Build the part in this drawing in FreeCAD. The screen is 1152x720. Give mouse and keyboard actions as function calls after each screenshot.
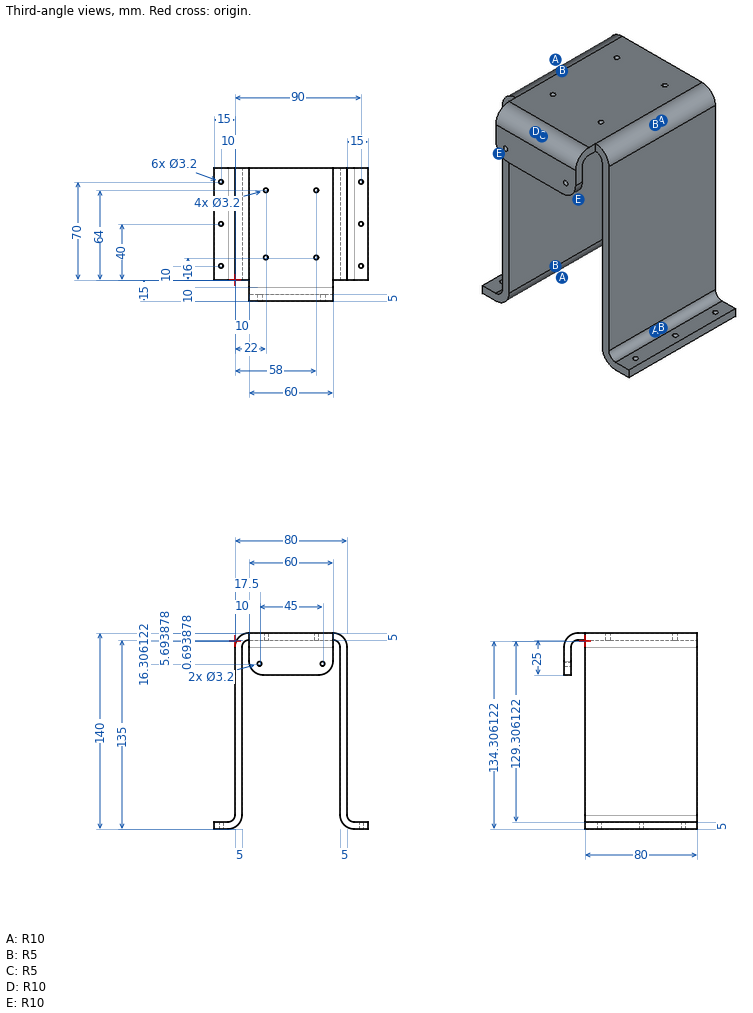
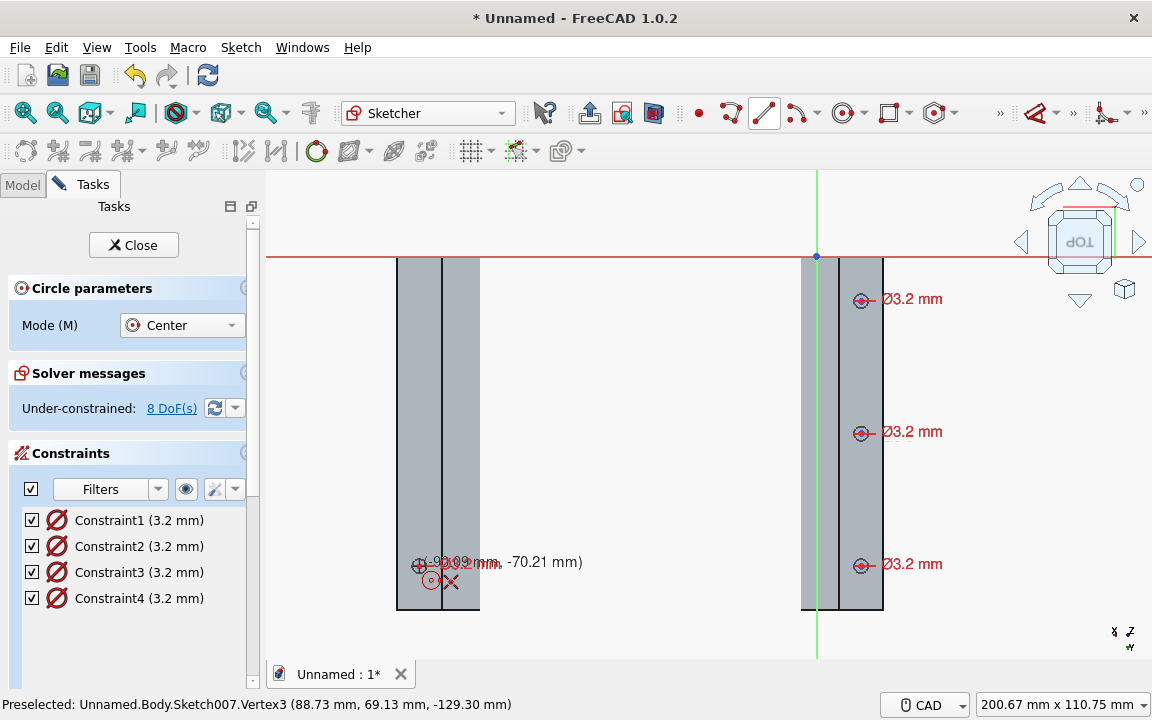
scroll(420, 433, up, 6)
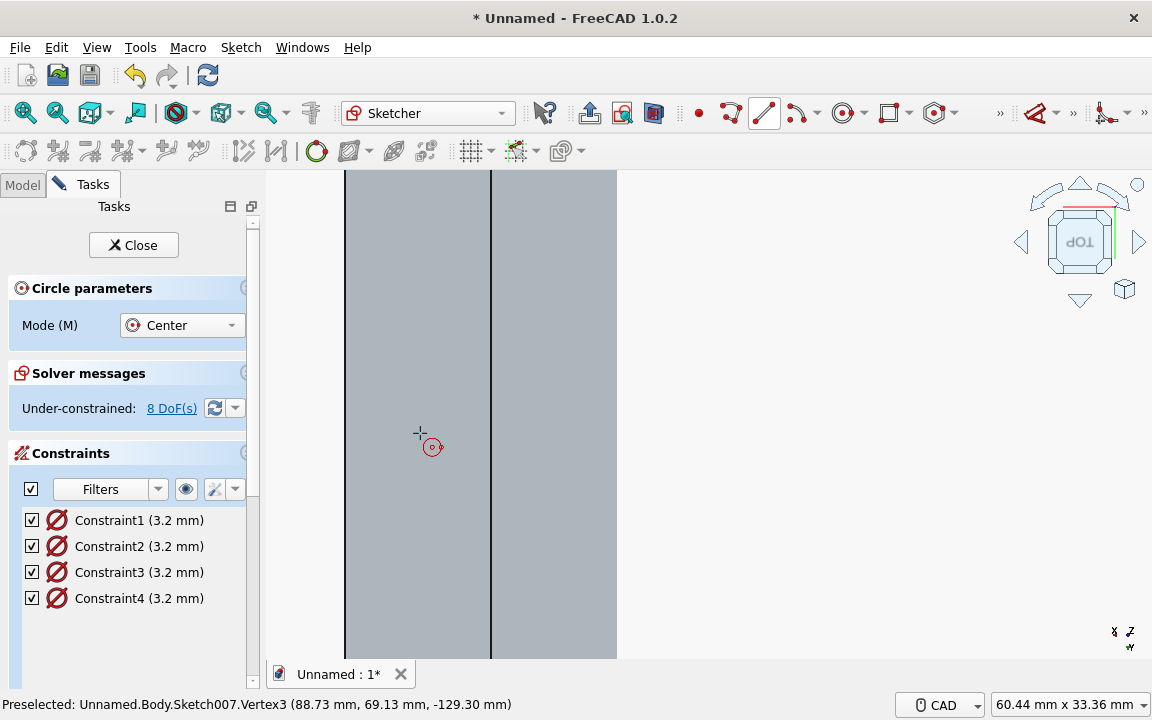
click(418, 433)
move(435, 417)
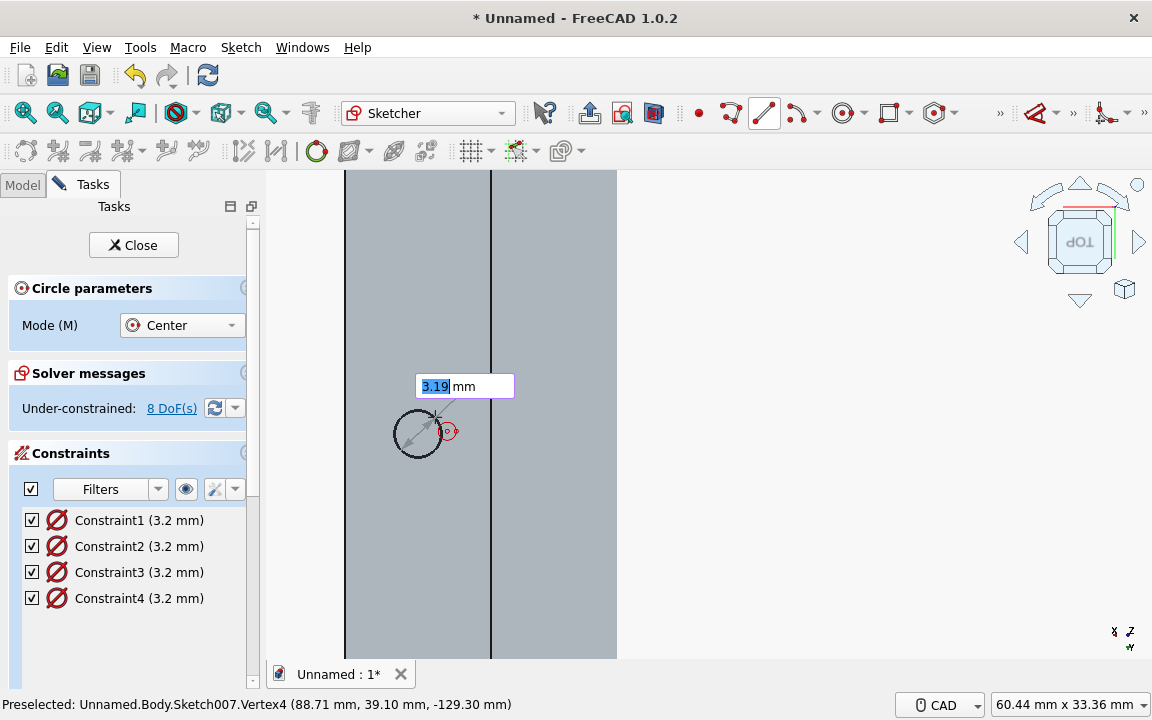
text(3.2)
key(Return)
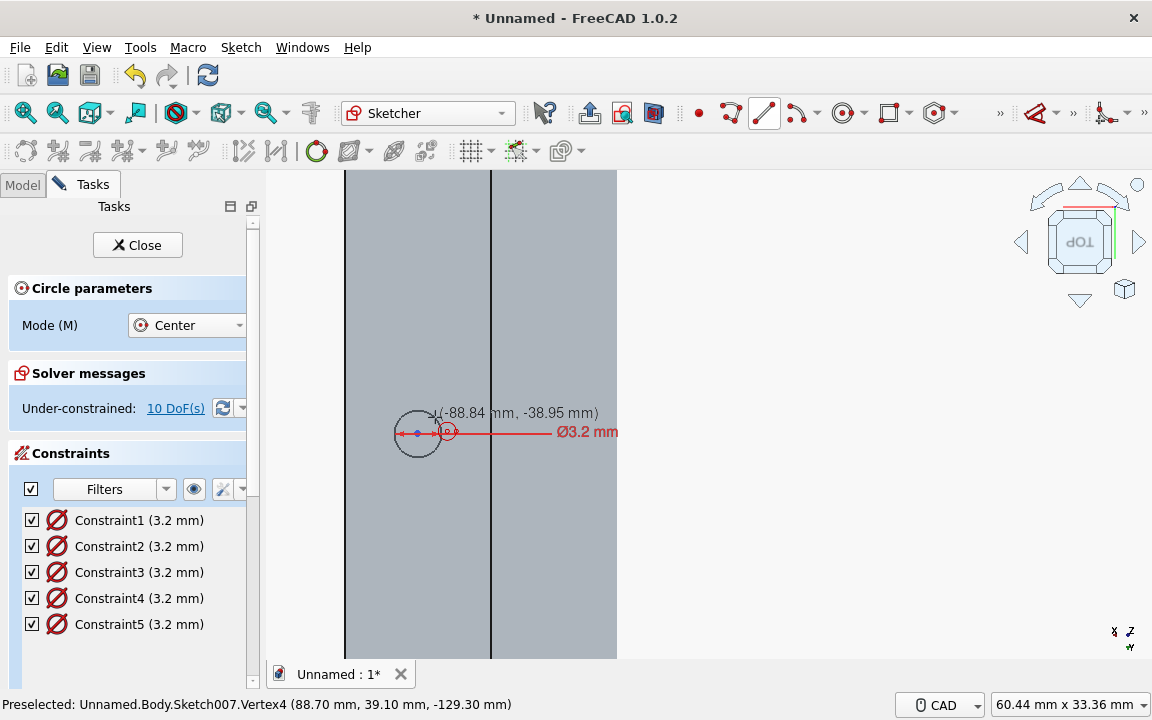
scroll(420, 433, down, 6)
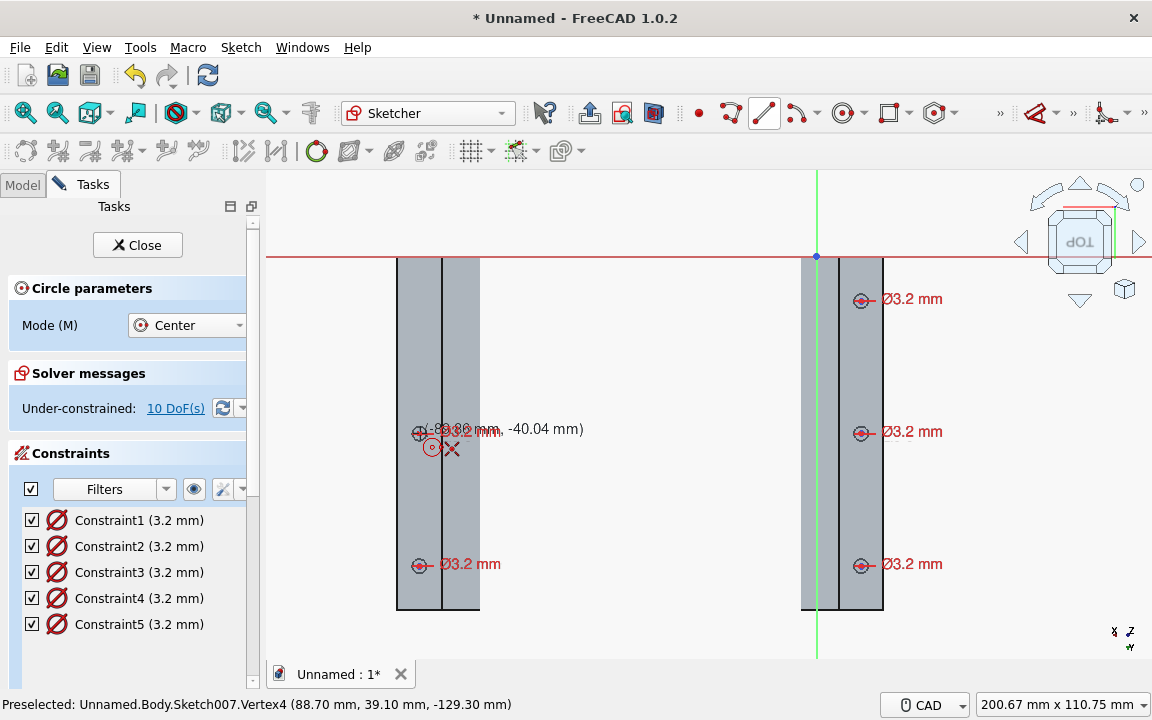
scroll(420, 301, up, 6)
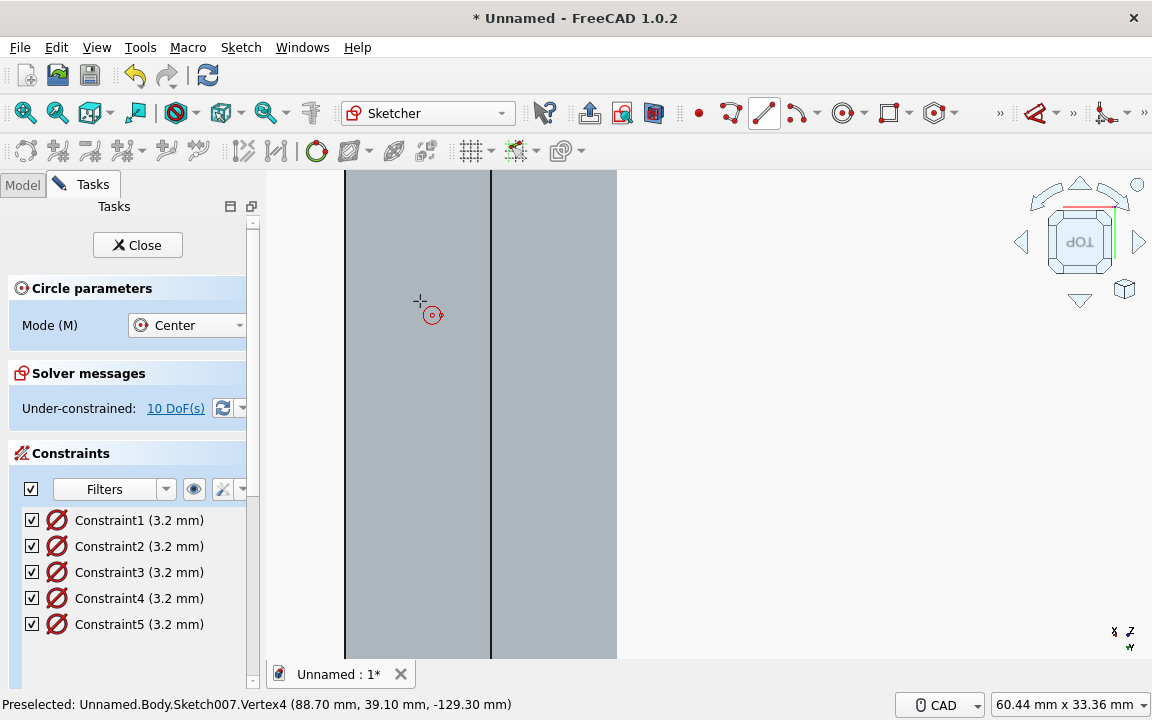
click(418, 300)
move(435, 284)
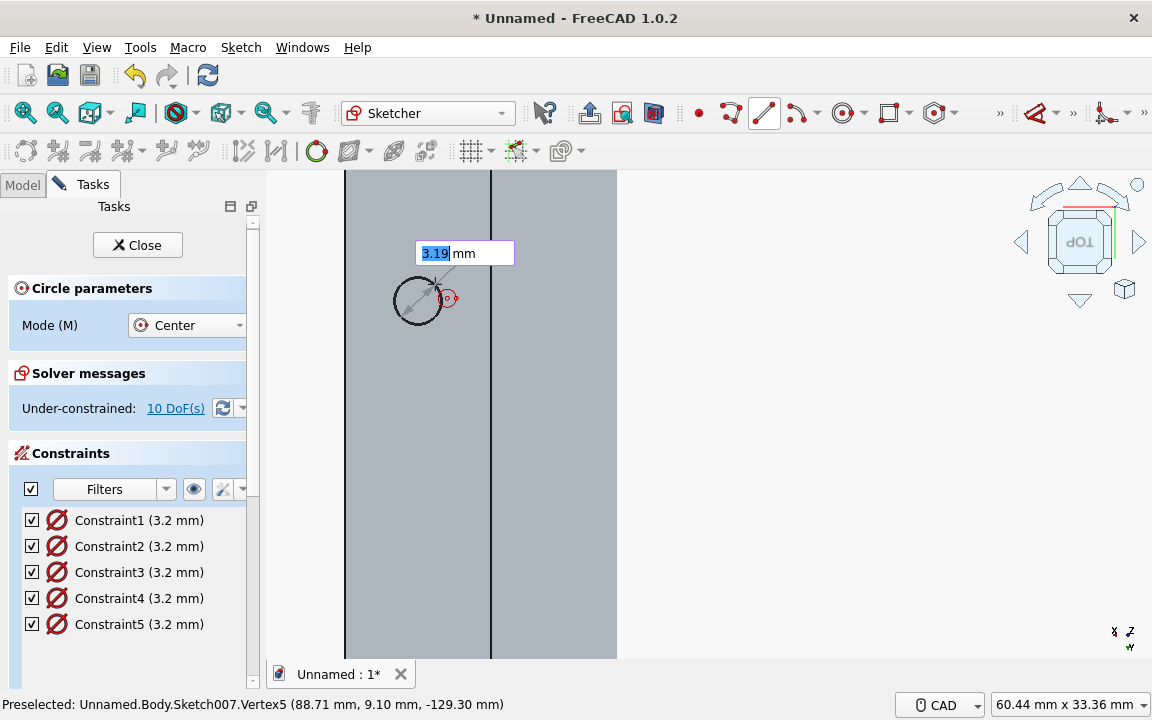
text(3.2)
key(Return)
key(Escape)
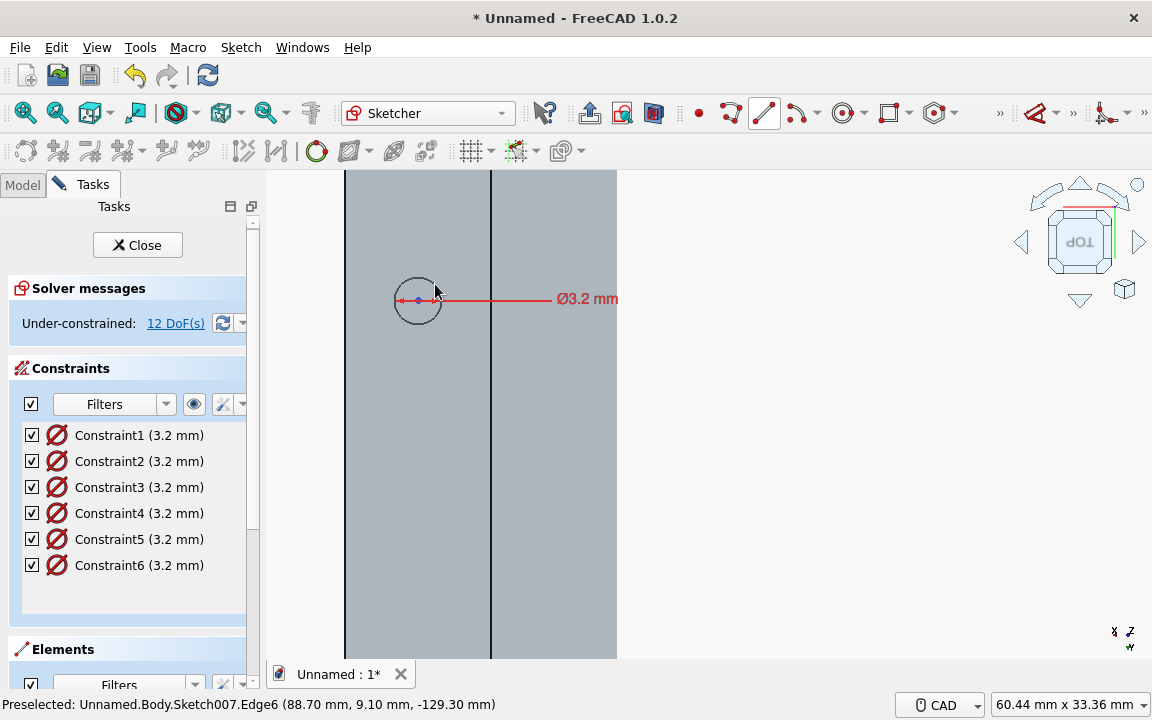
click(1036, 114)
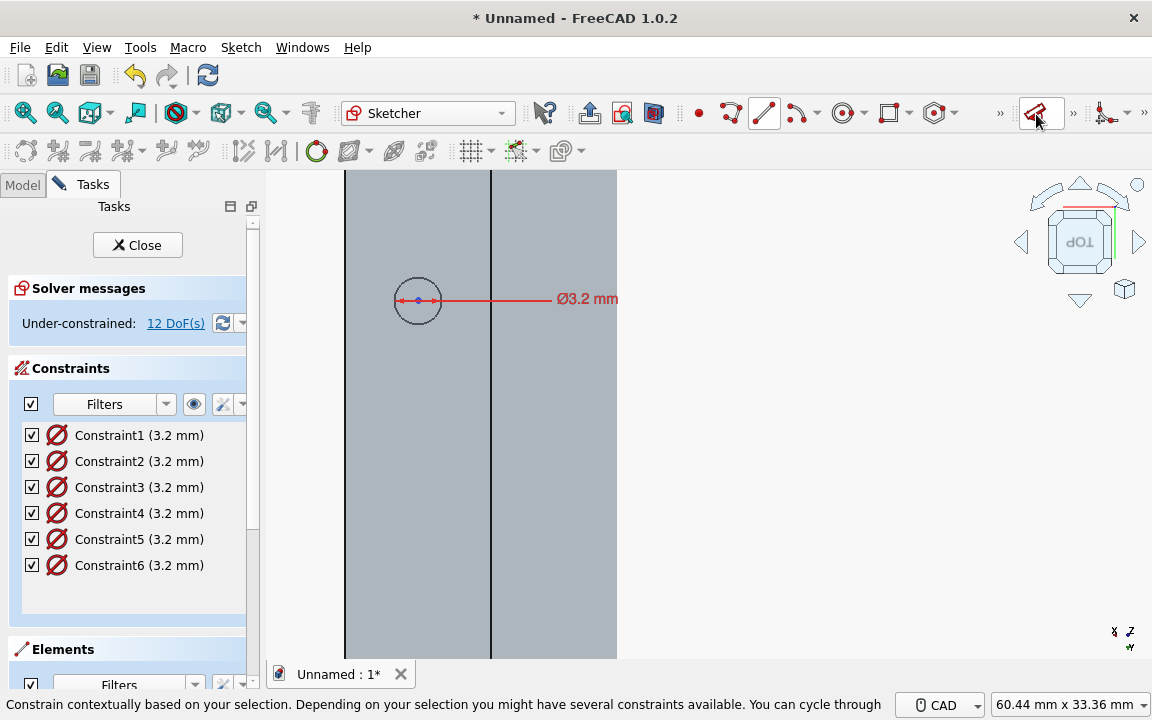
scroll(420, 301, down, 6)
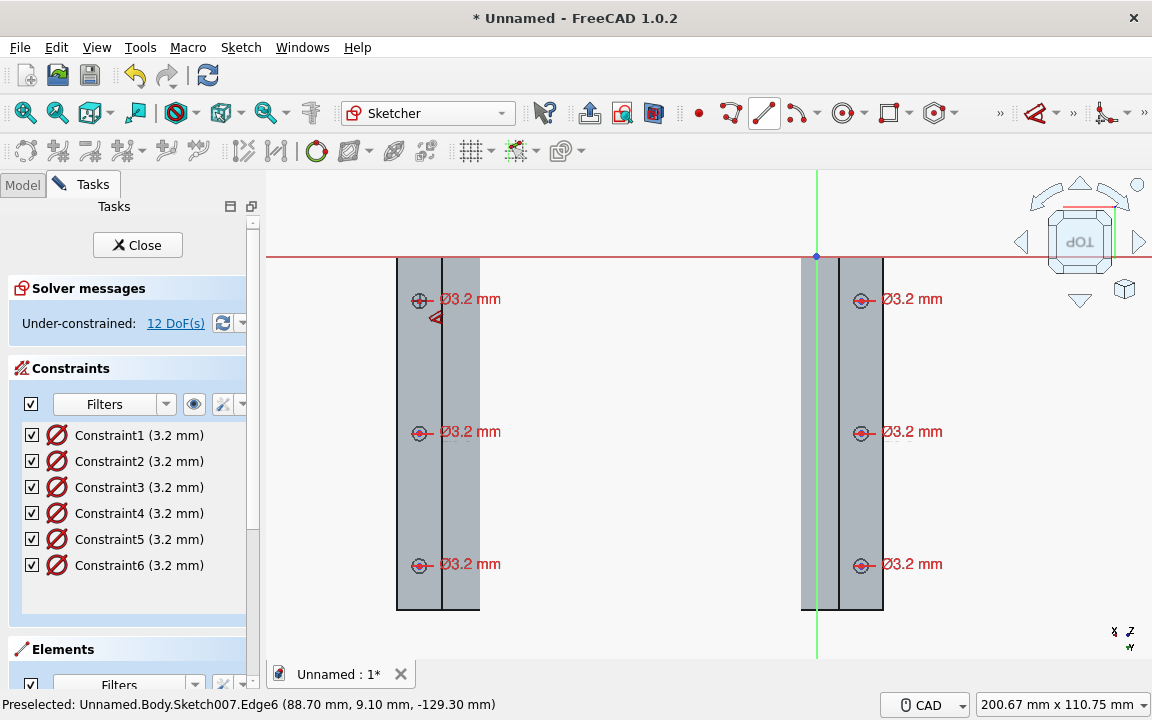
click(861, 566)
click(839, 223)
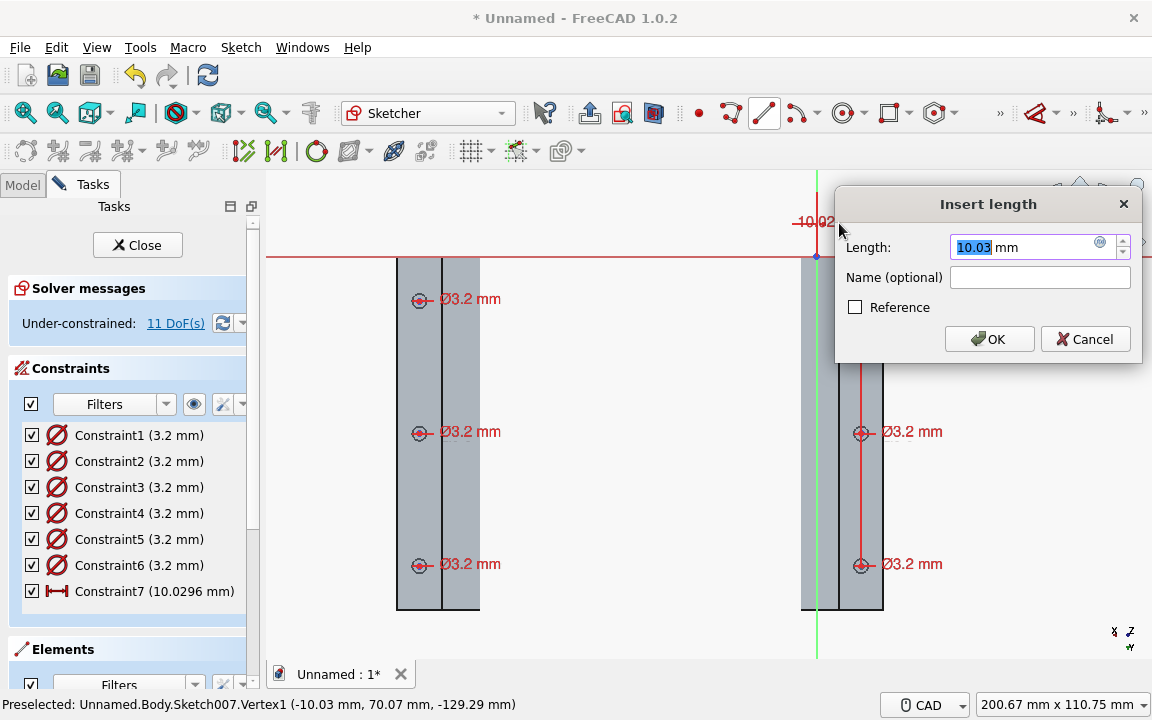
text(10)
key(Return)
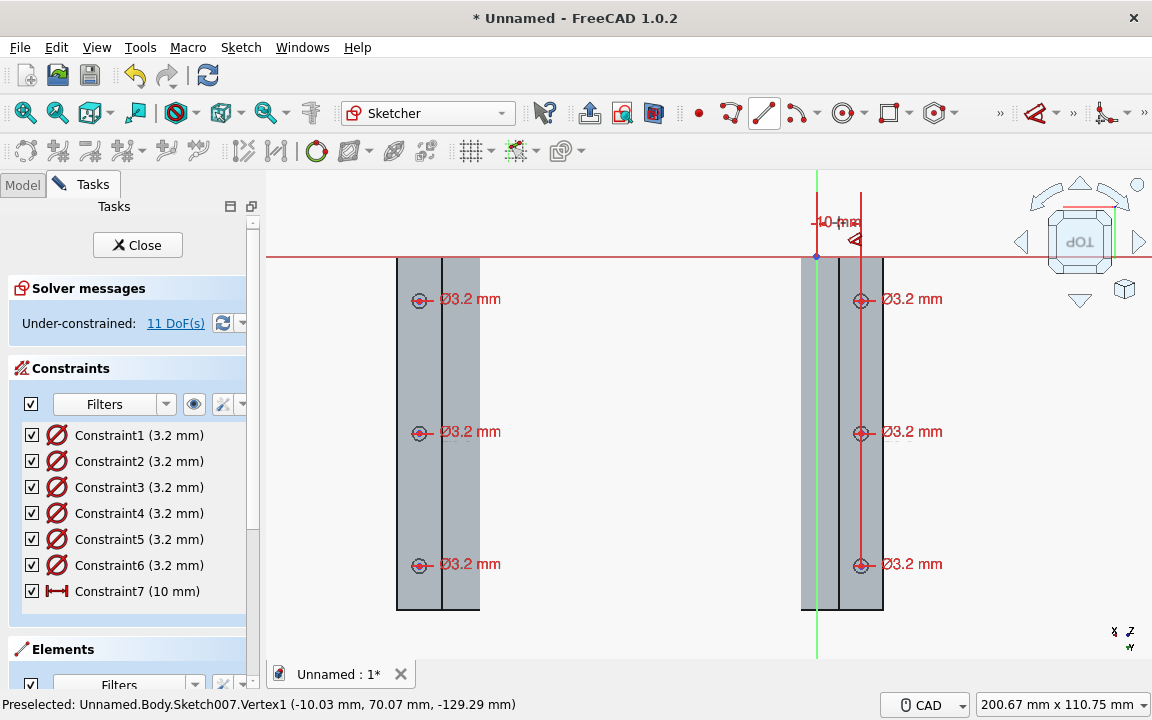
click(861, 566)
click(895, 412)